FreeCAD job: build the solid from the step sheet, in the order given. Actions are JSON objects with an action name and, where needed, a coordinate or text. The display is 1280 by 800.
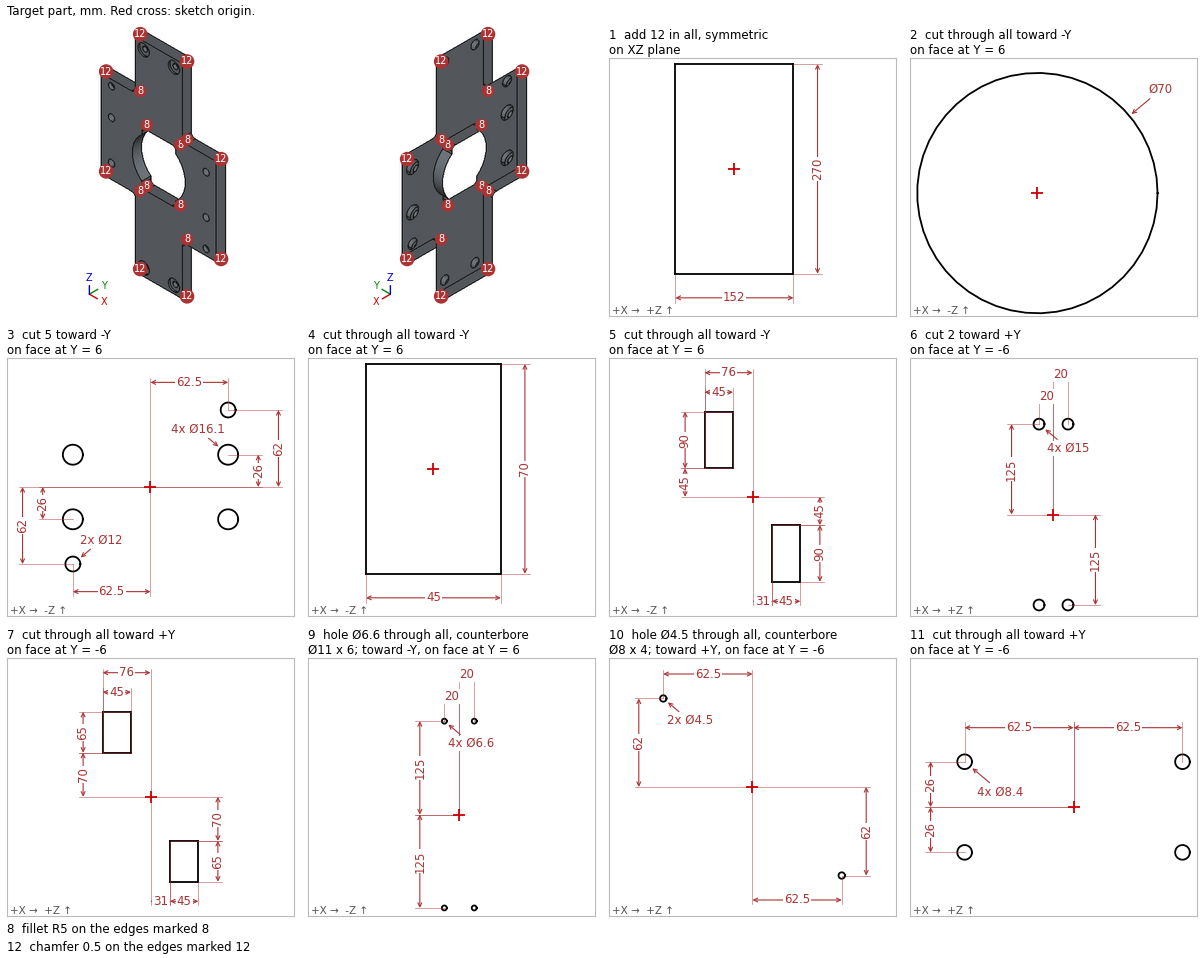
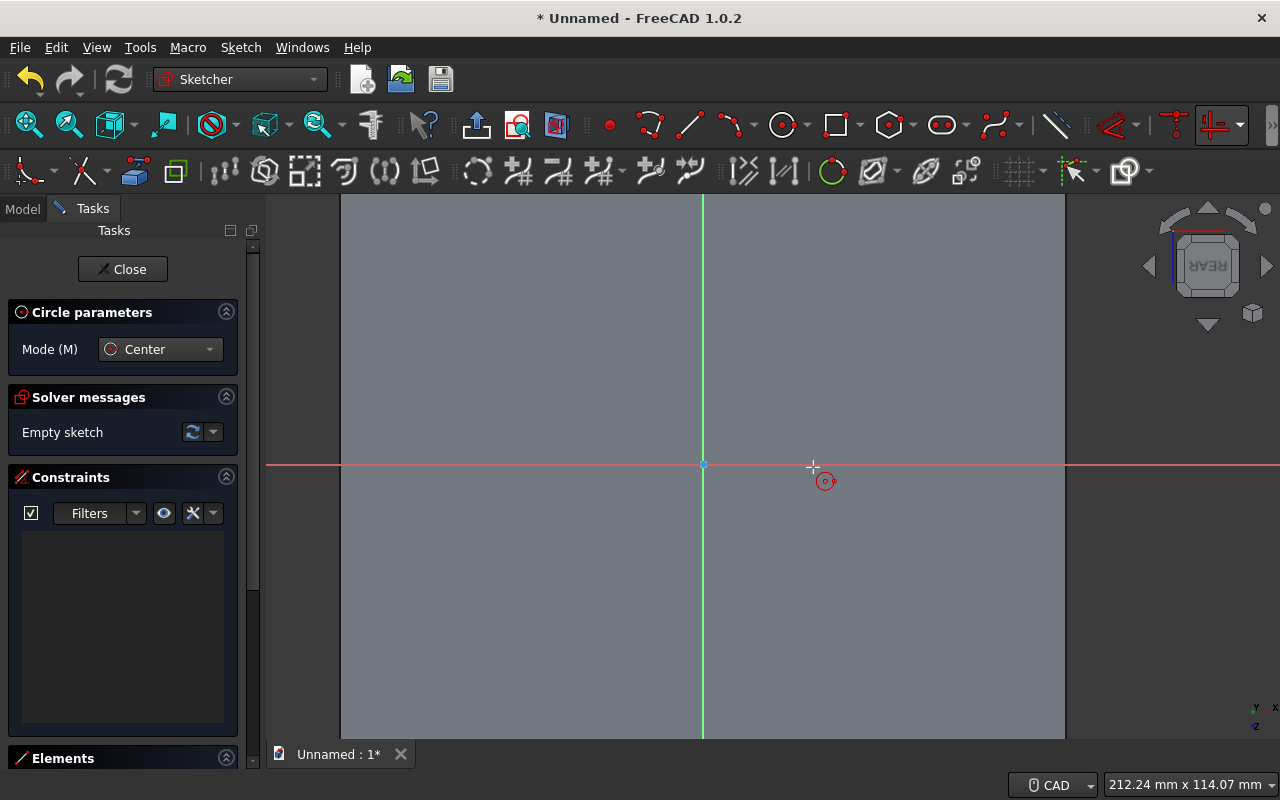
{"action": "left_click", "coordinate": [703, 465]}
{"action": "mouse_move", "coordinate": [822, 347]}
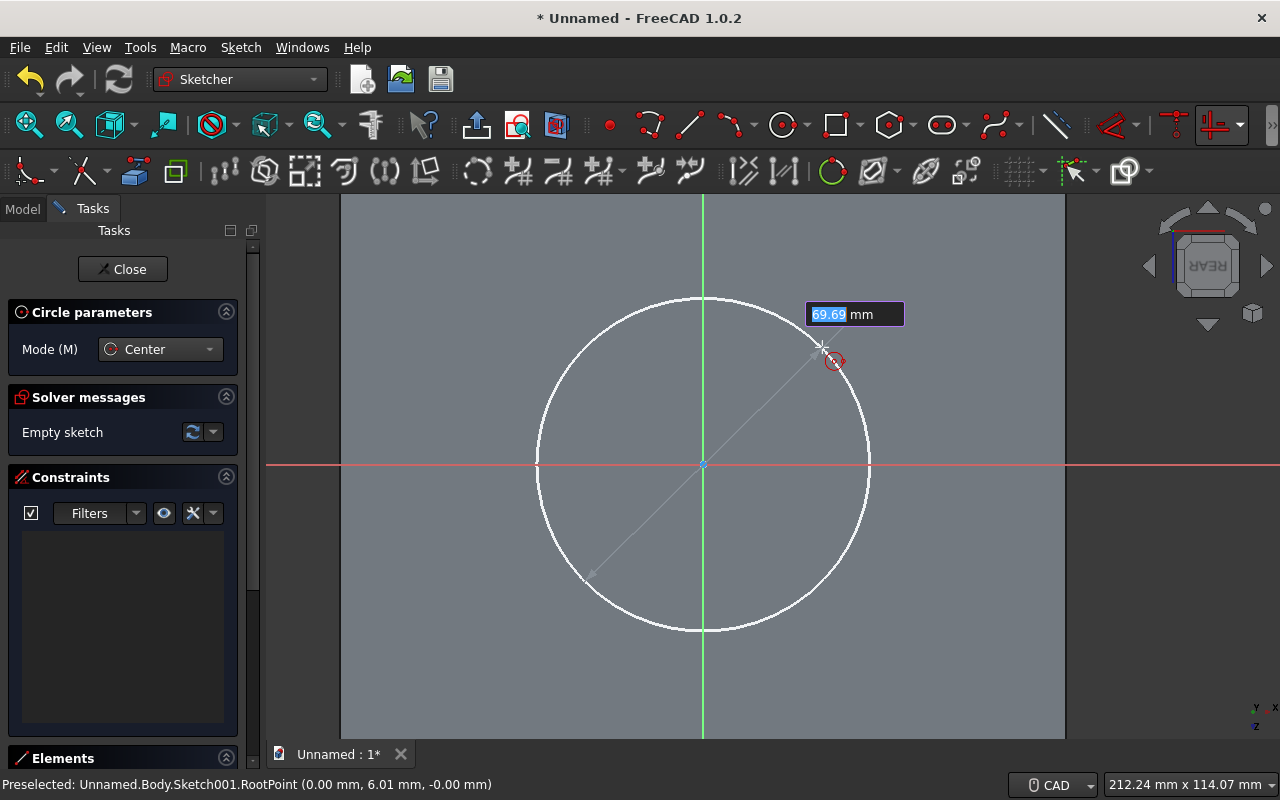
{"action": "type", "text": "70"}
{"action": "key", "text": "Return"}
{"action": "key", "text": "Escape"}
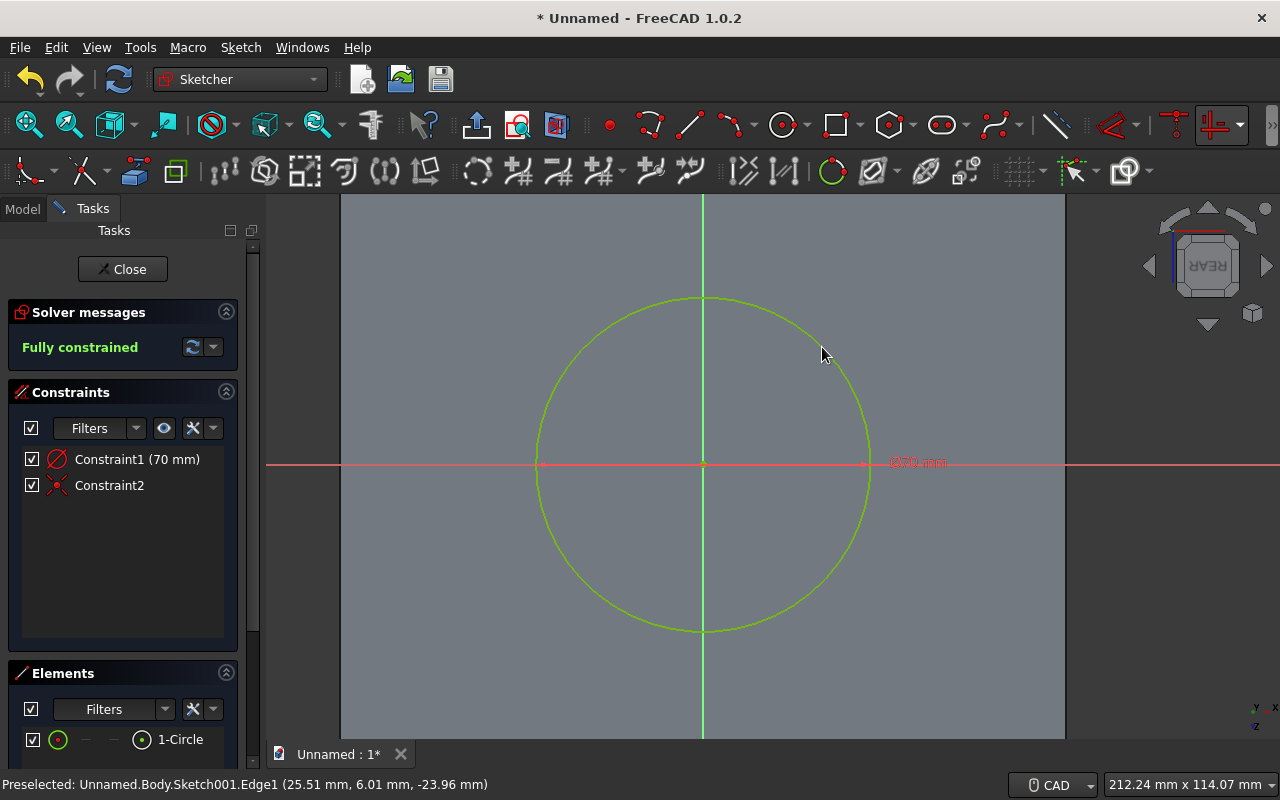
{"action": "left_click", "coordinate": [123, 269]}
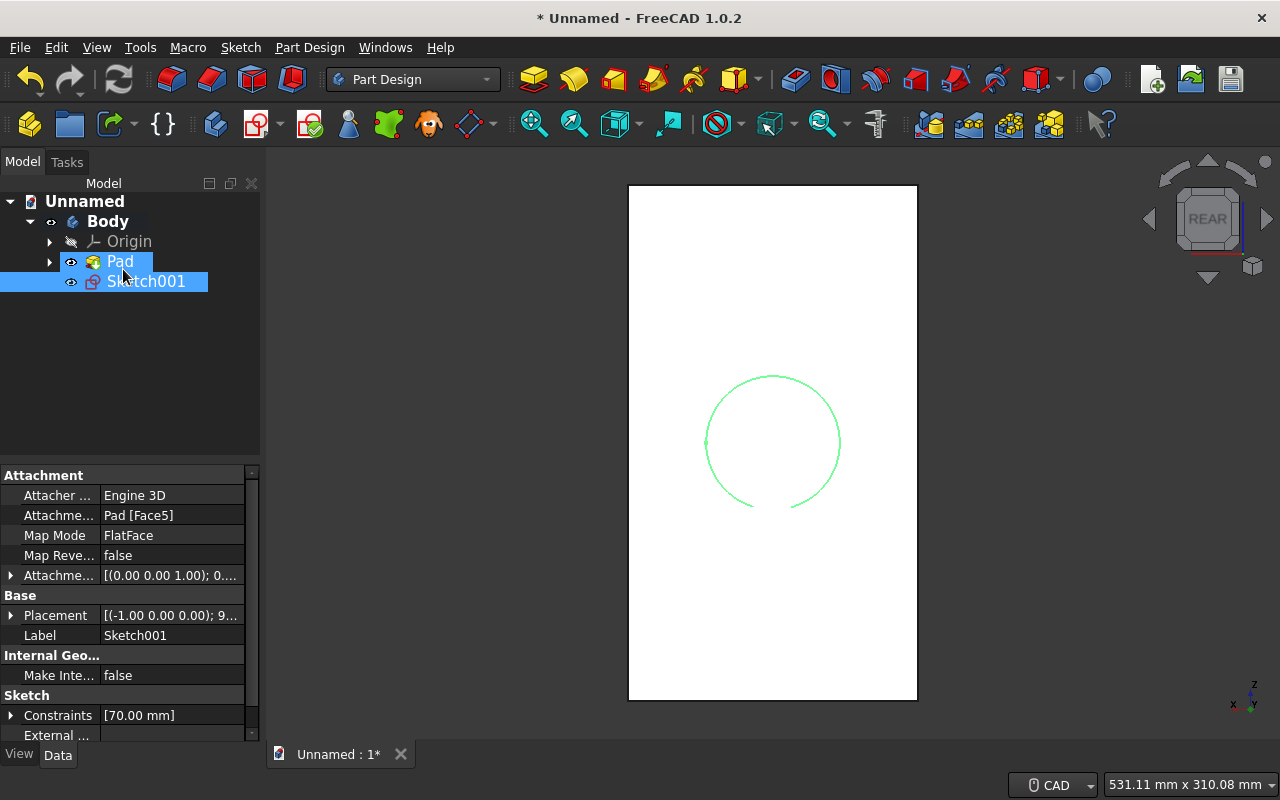
{"action": "left_click", "coordinate": [796, 80]}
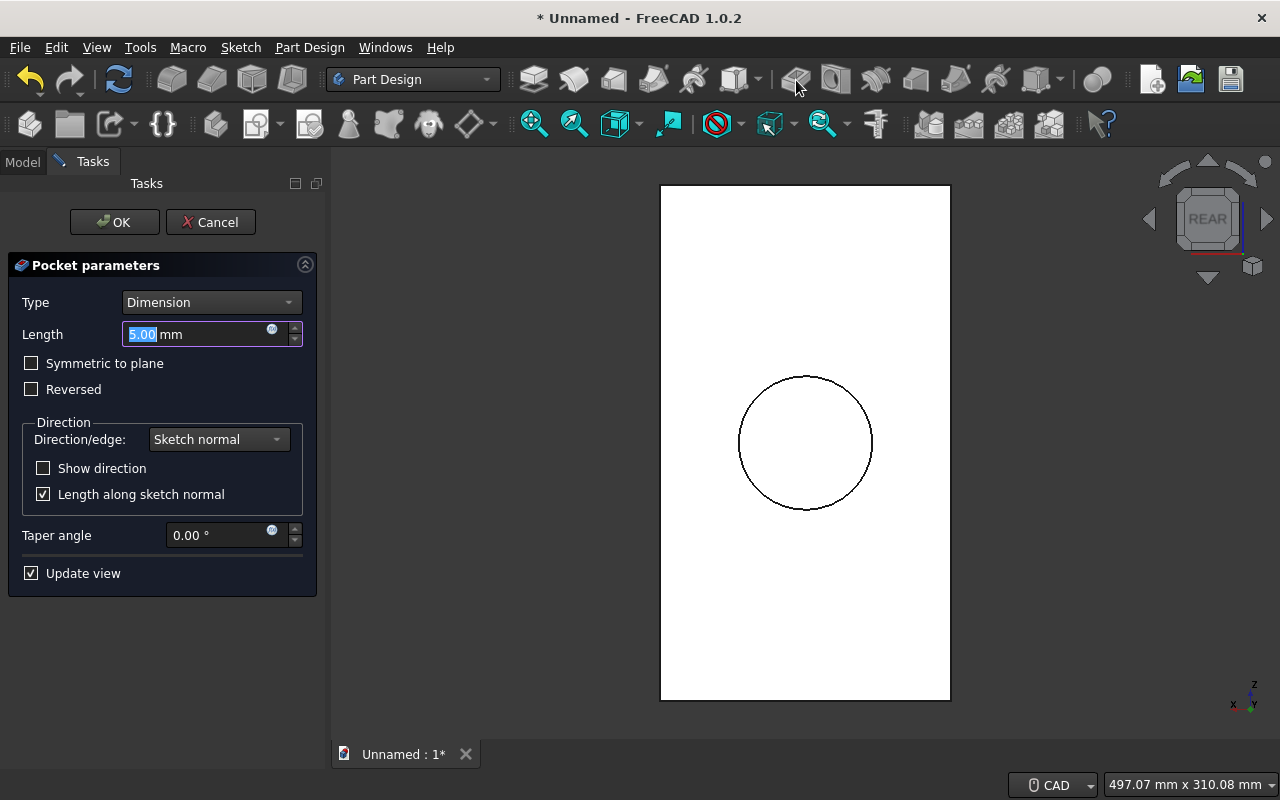
{"action": "left_click", "coordinate": [212, 302]}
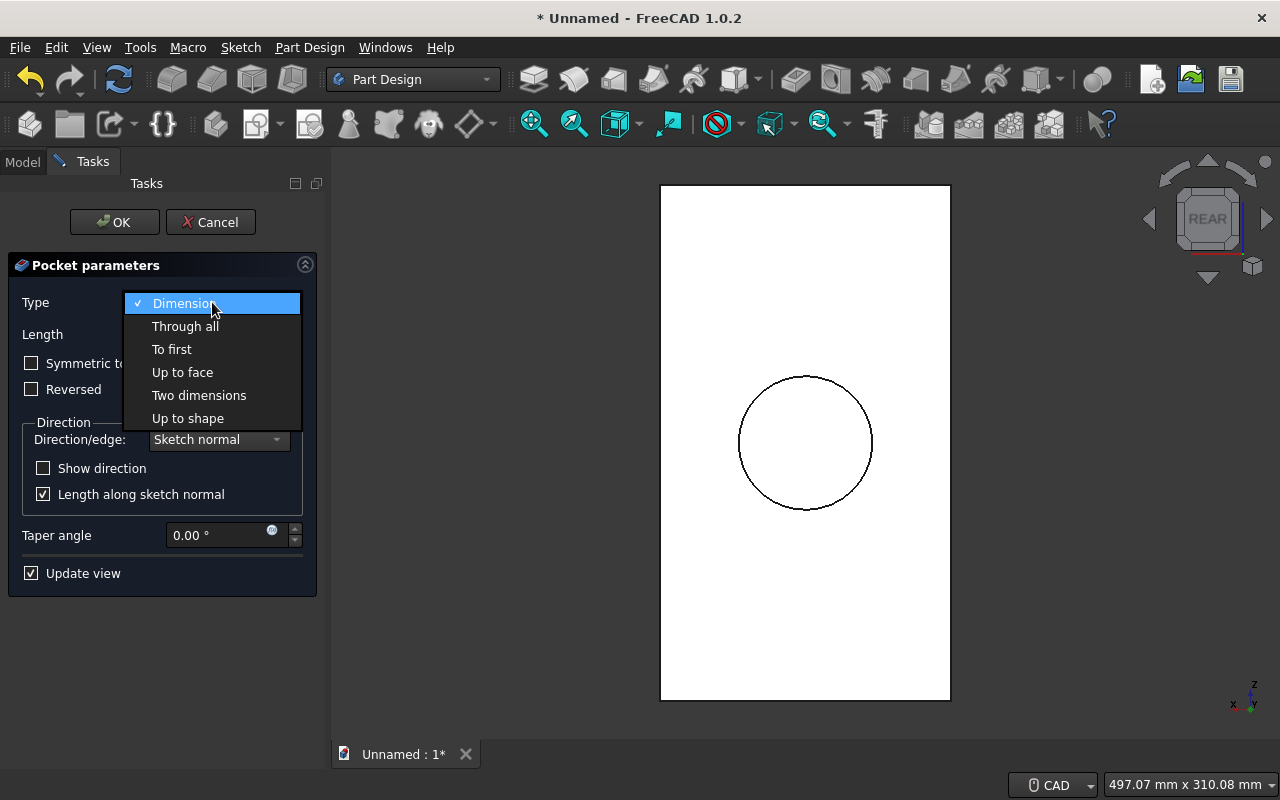
{"action": "left_click", "coordinate": [212, 326]}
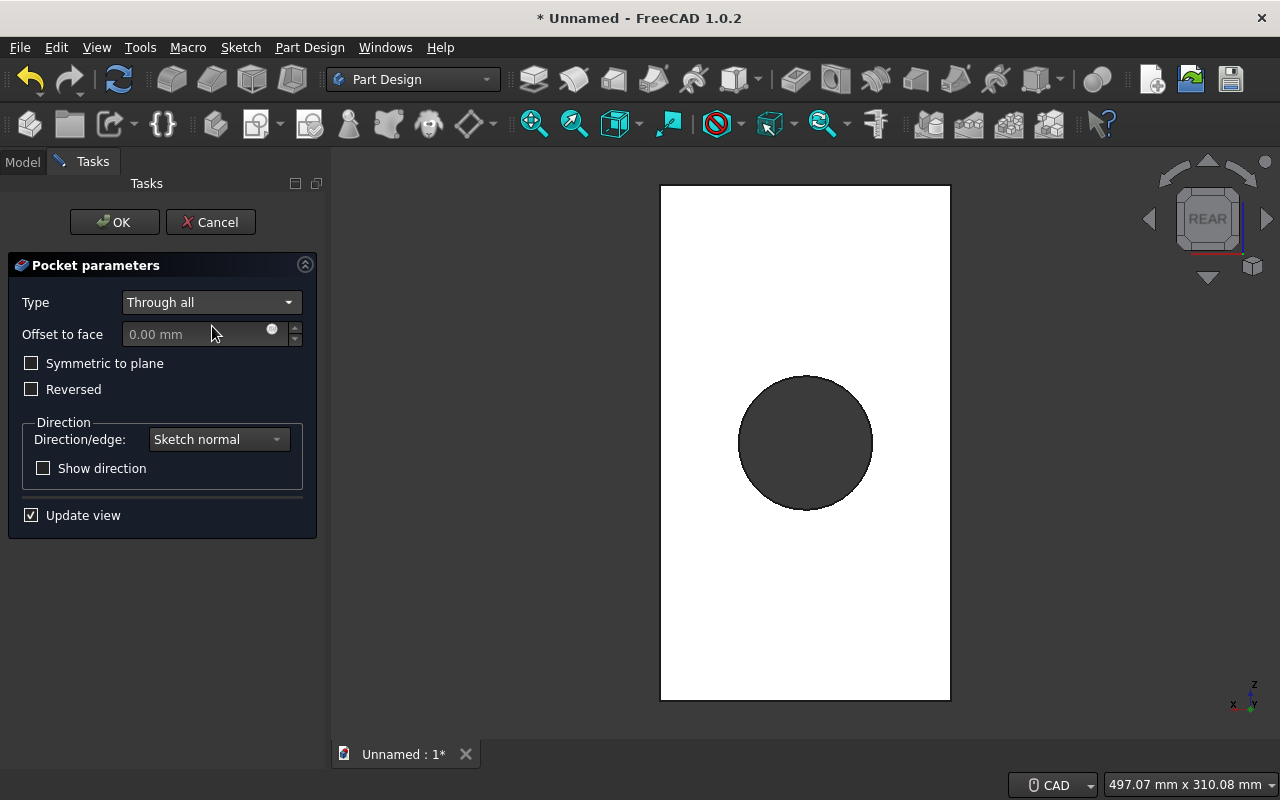
{"action": "left_click", "coordinate": [115, 222]}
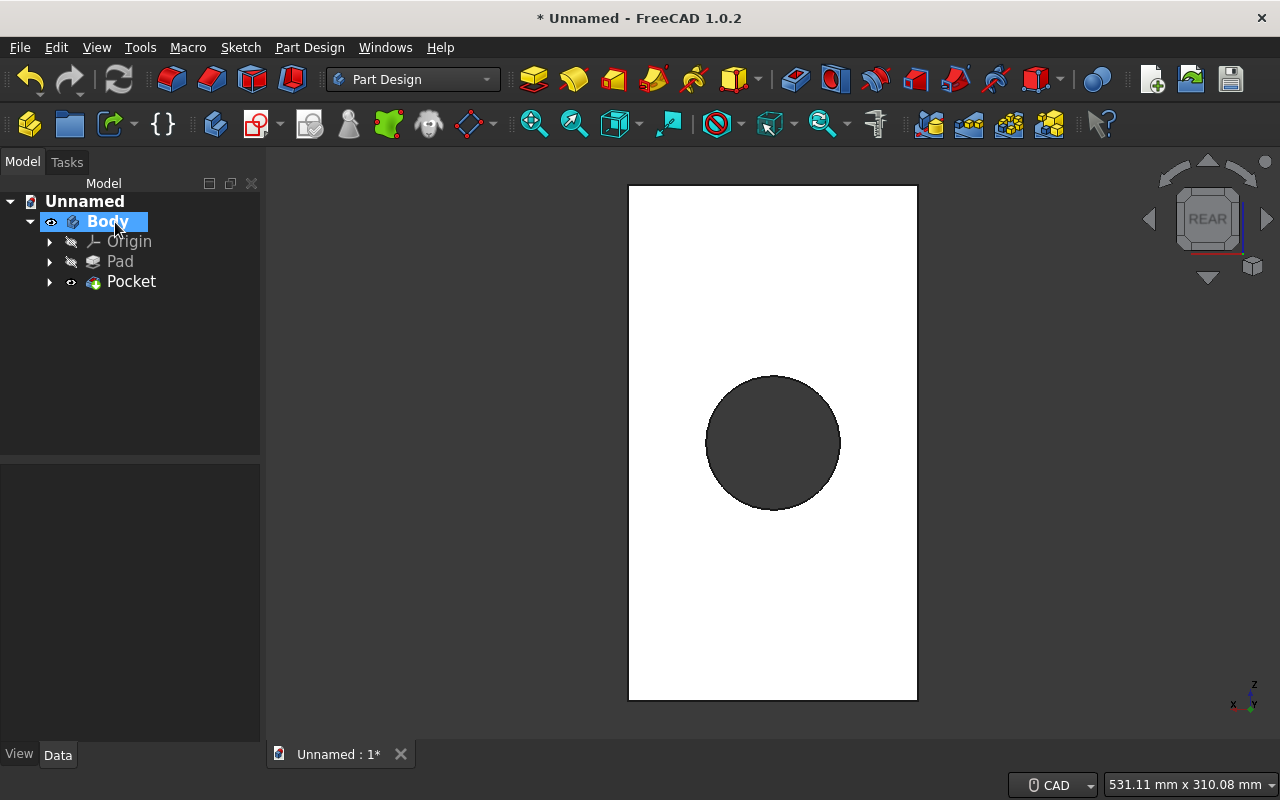
{"action": "left_click", "coordinate": [732, 295]}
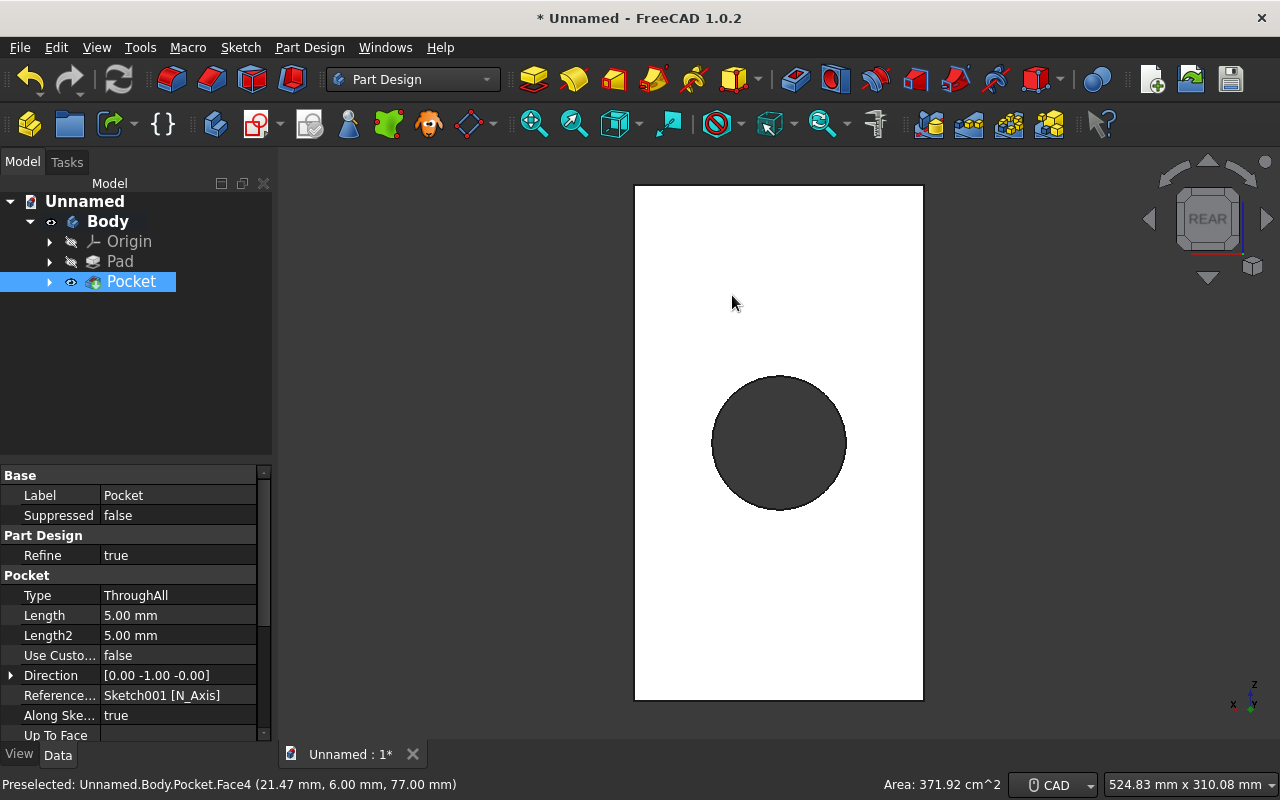
{"action": "left_click", "coordinate": [256, 124]}